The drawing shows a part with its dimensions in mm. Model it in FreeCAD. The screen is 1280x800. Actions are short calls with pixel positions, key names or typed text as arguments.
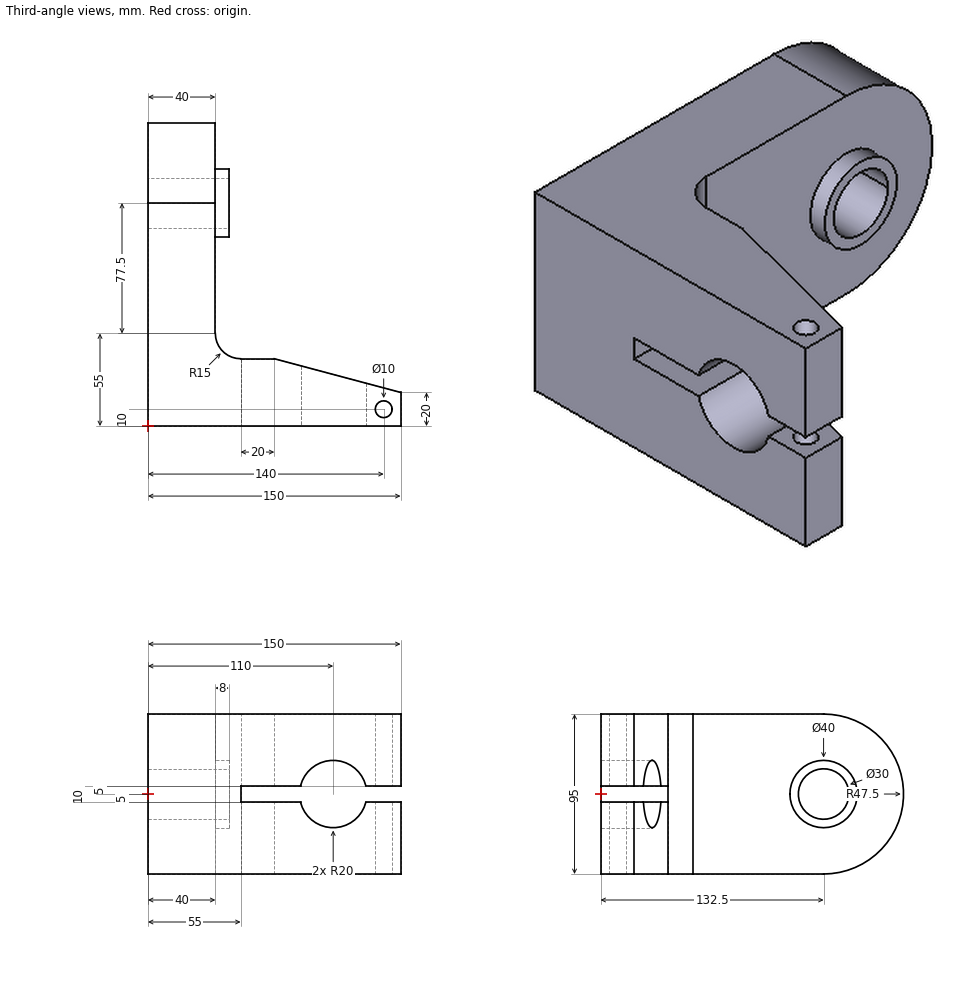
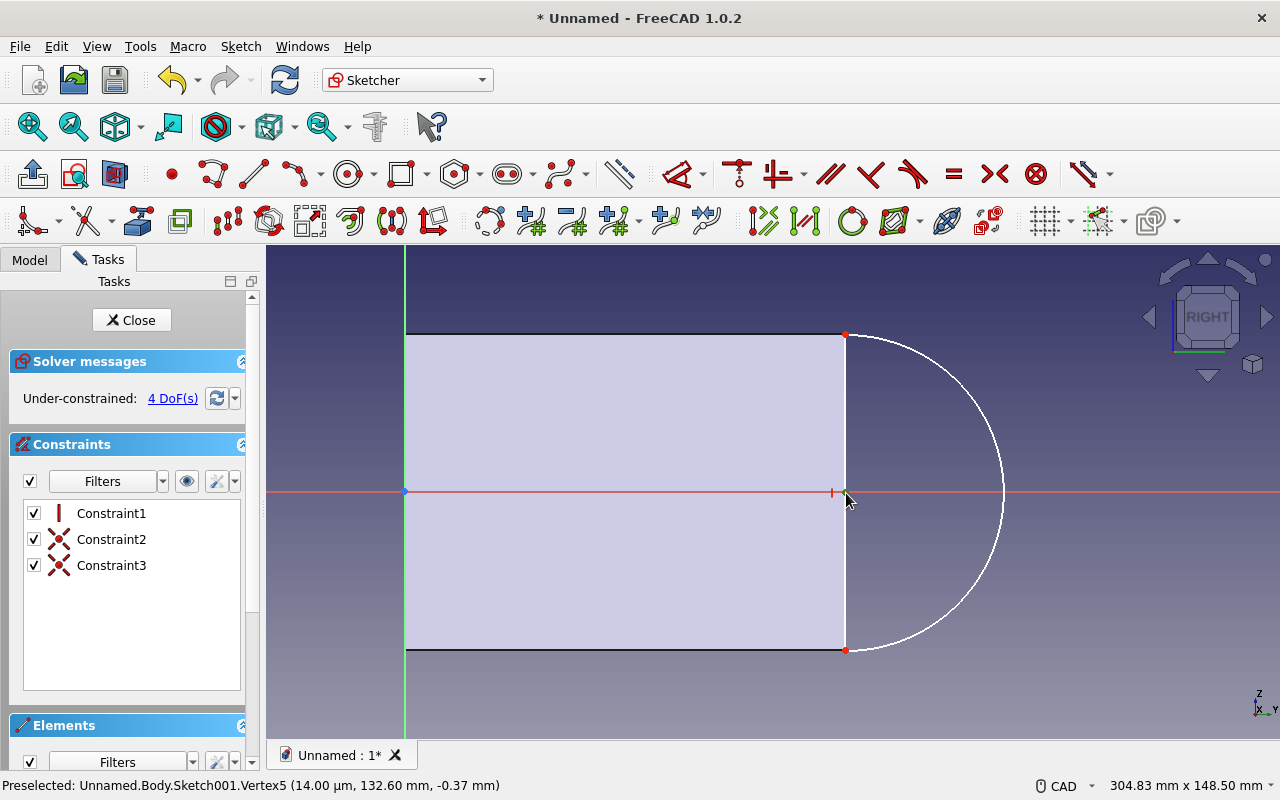
click(353, 492)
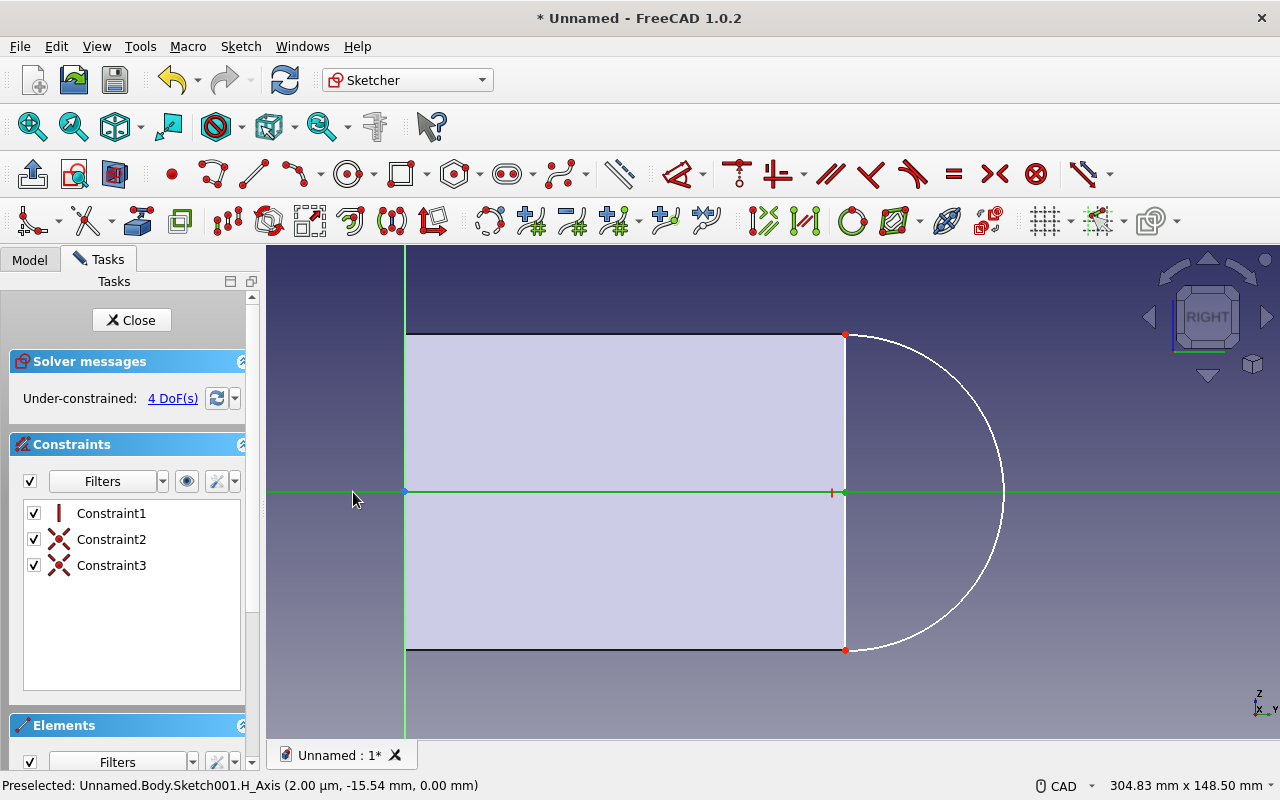
click(737, 174)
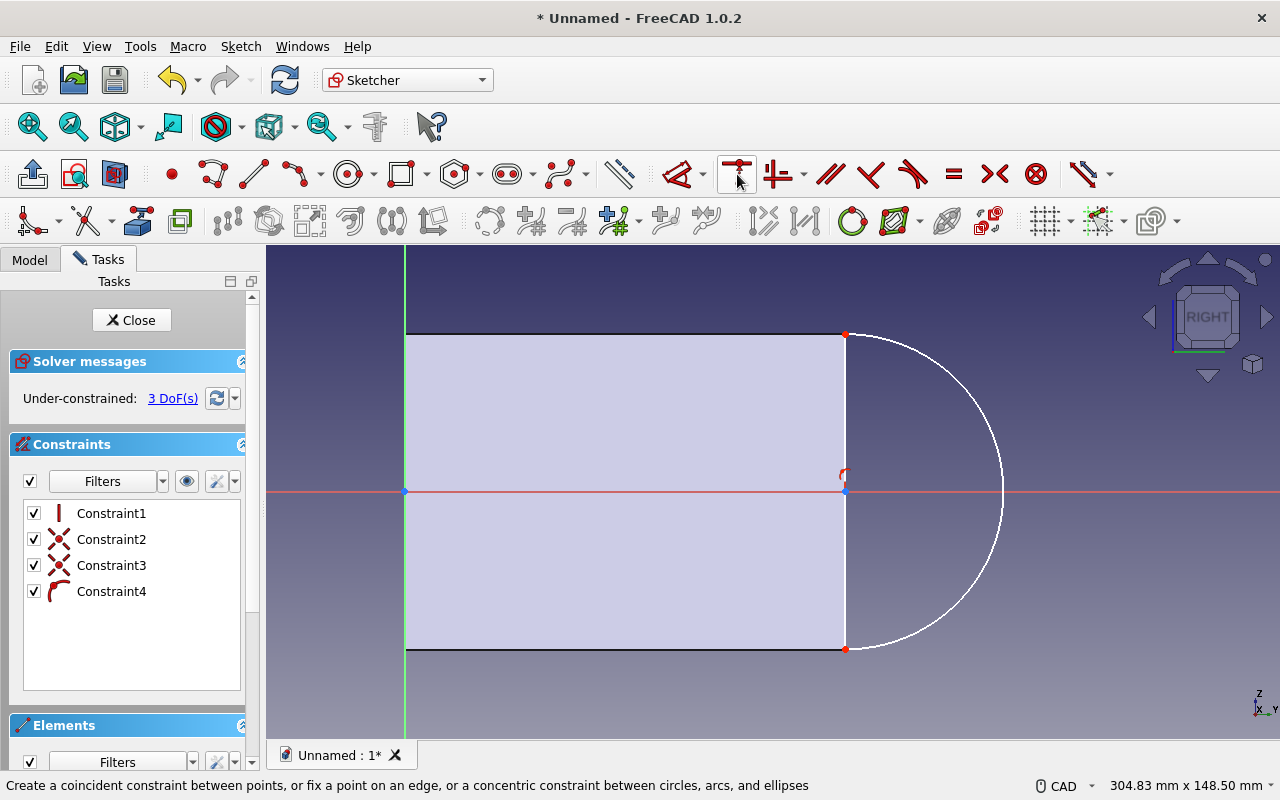
click(676, 174)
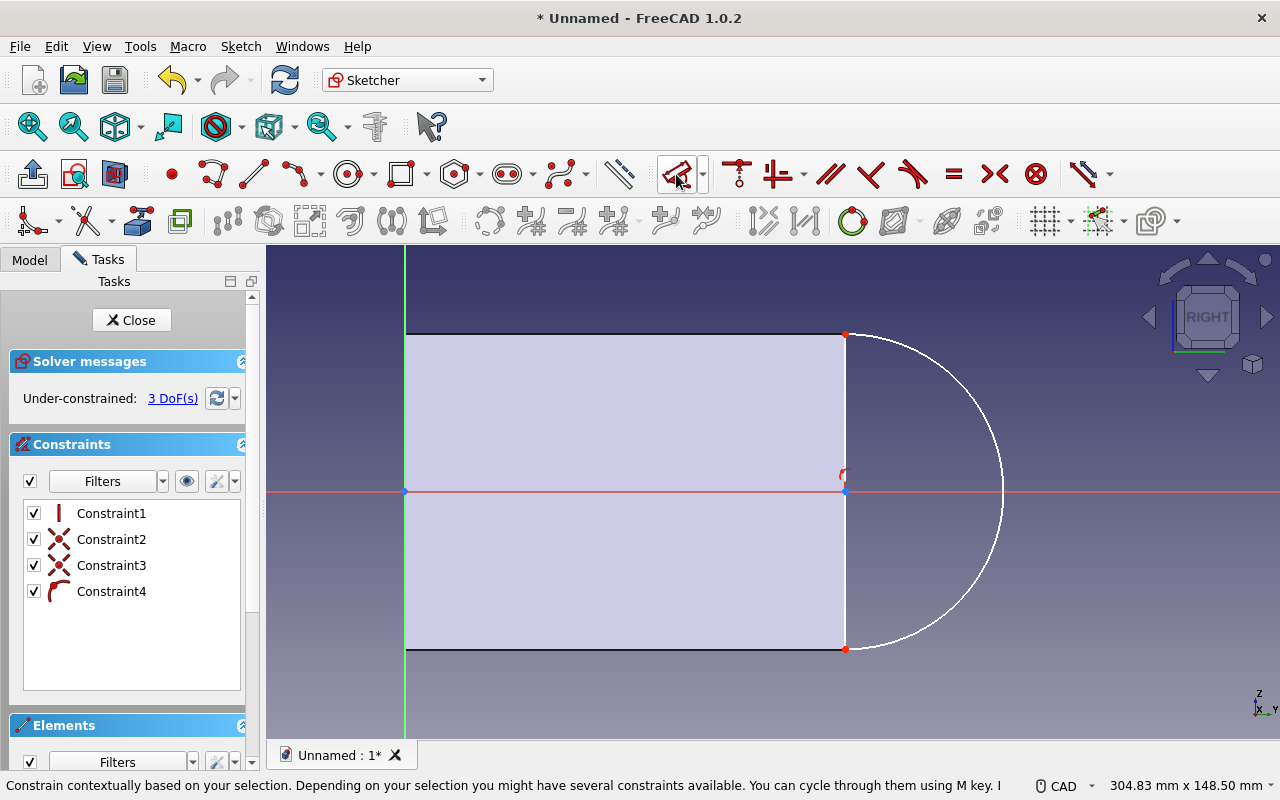
click(973, 585)
click(999, 604)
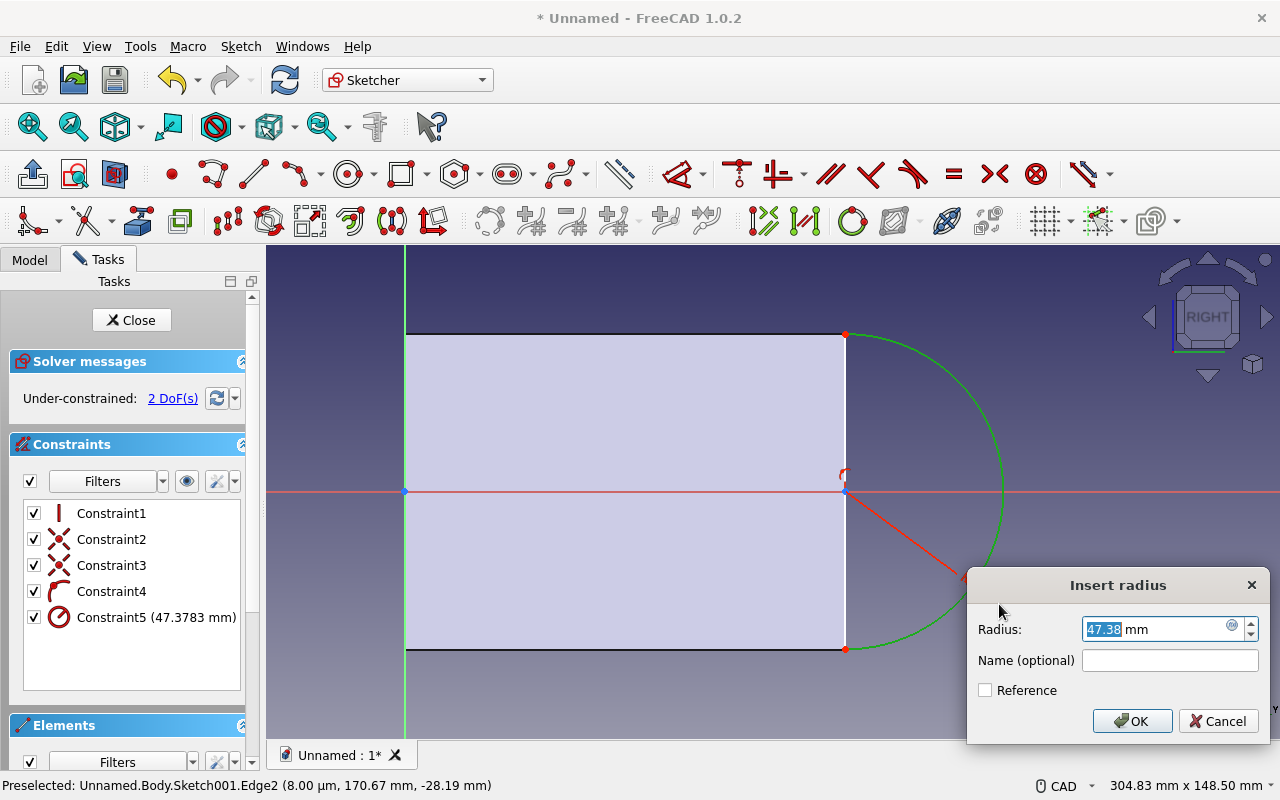
text(47.5)
key(Return)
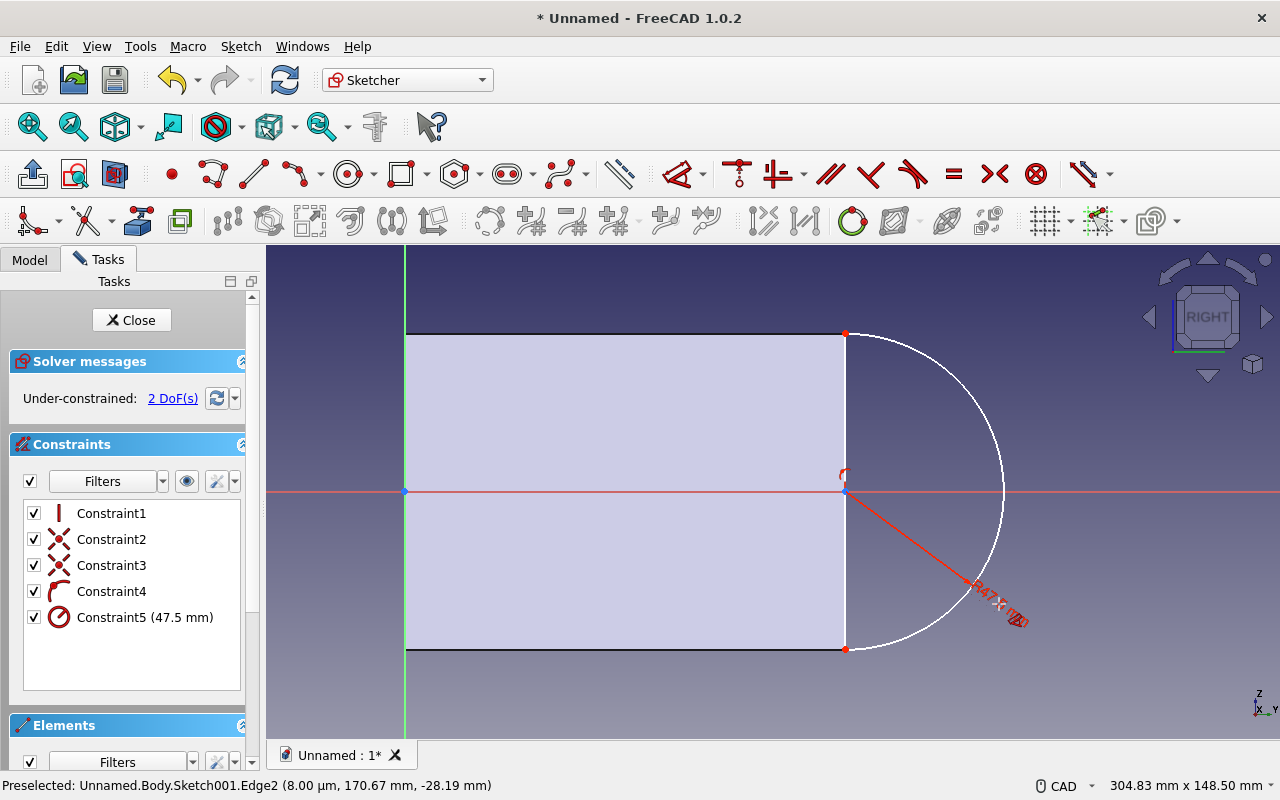
click(845, 650)
click(625, 684)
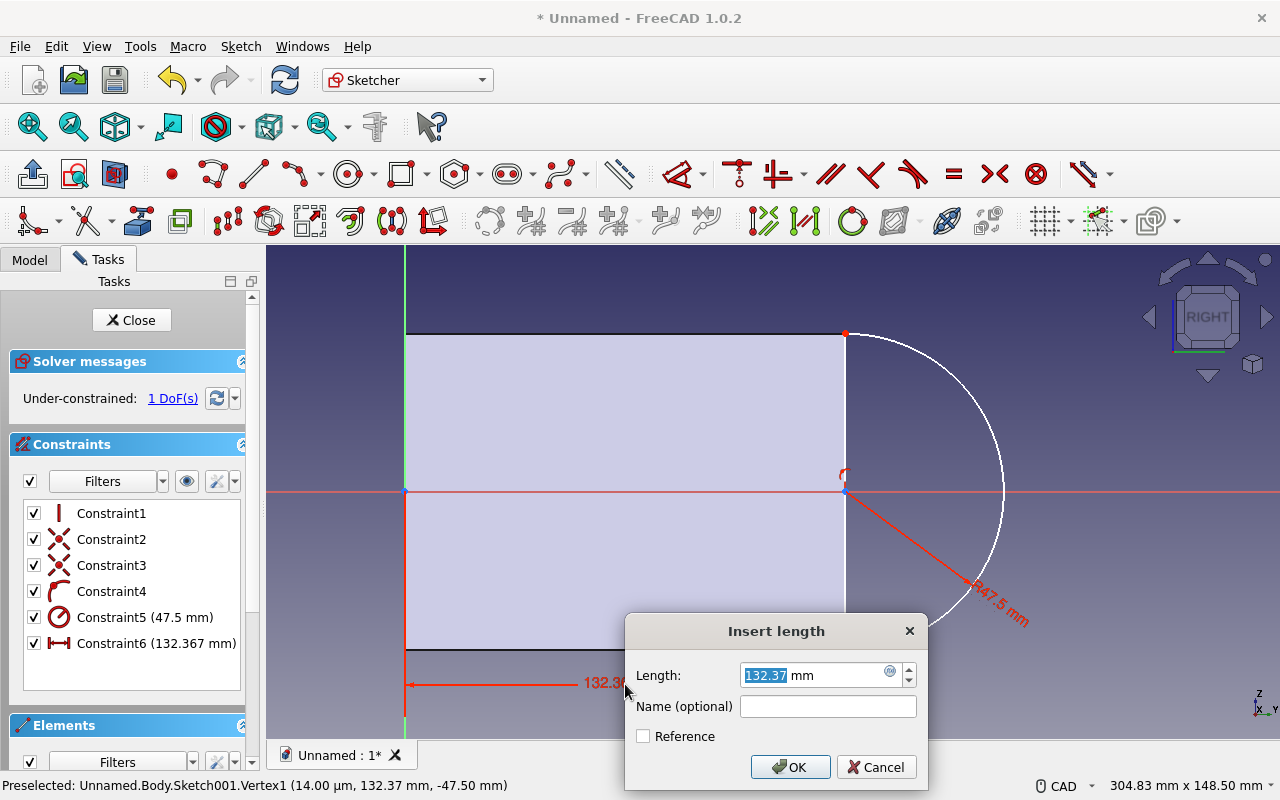
text(132.5)
key(Return)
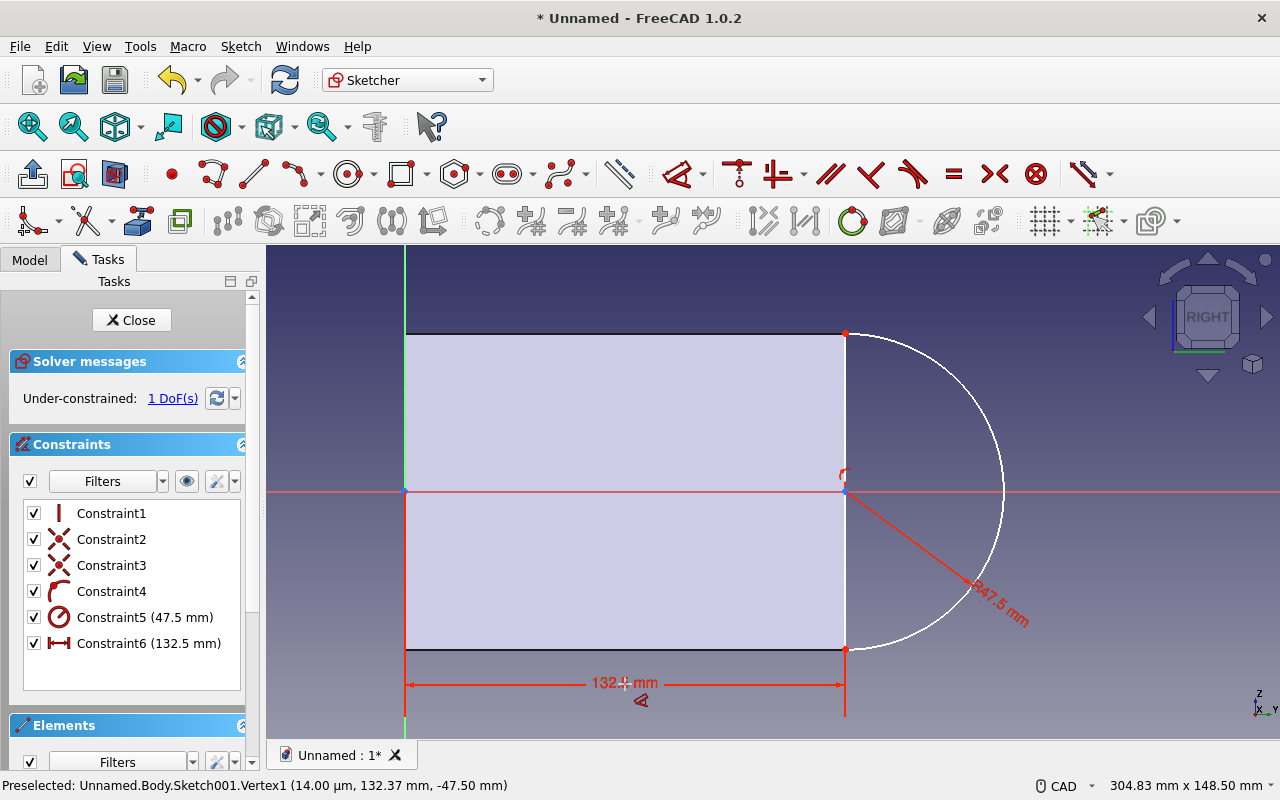
click(846, 492)
click(625, 526)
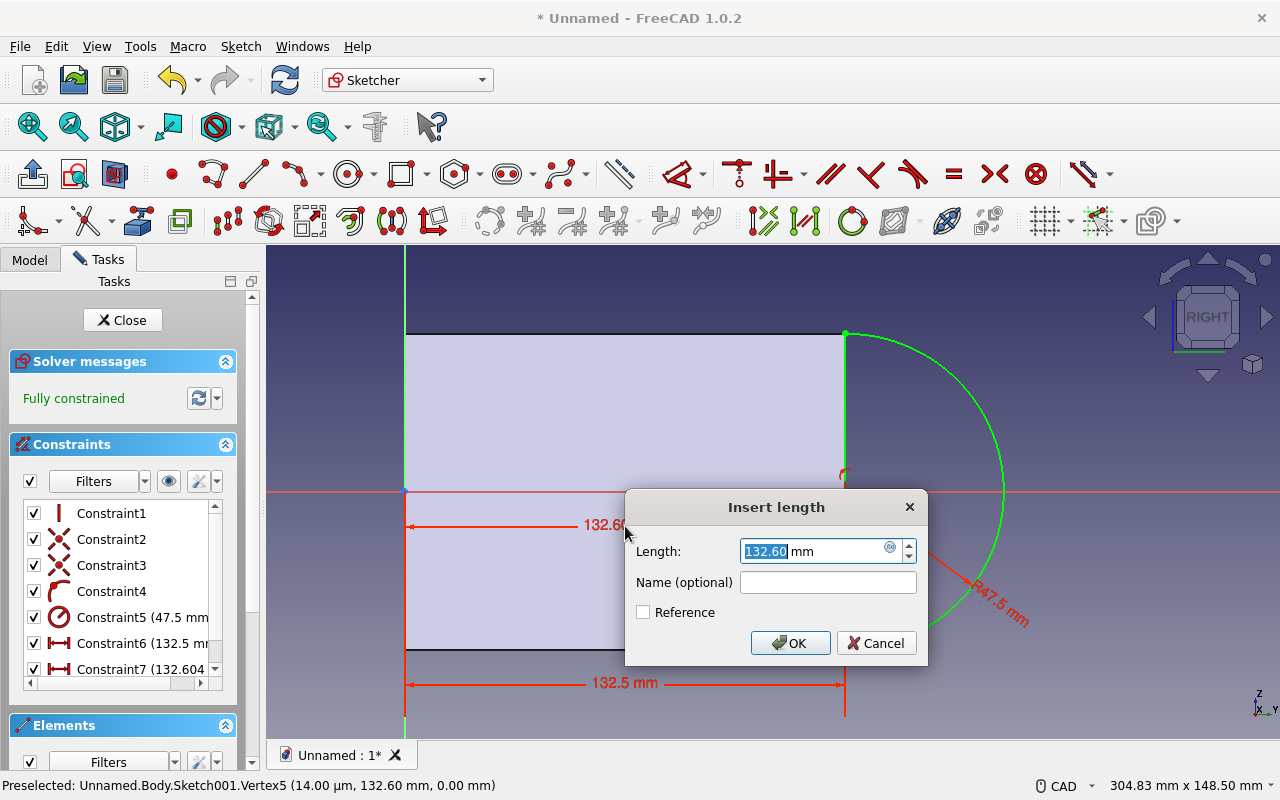
text(132.5)
key(Return)
key(Escape)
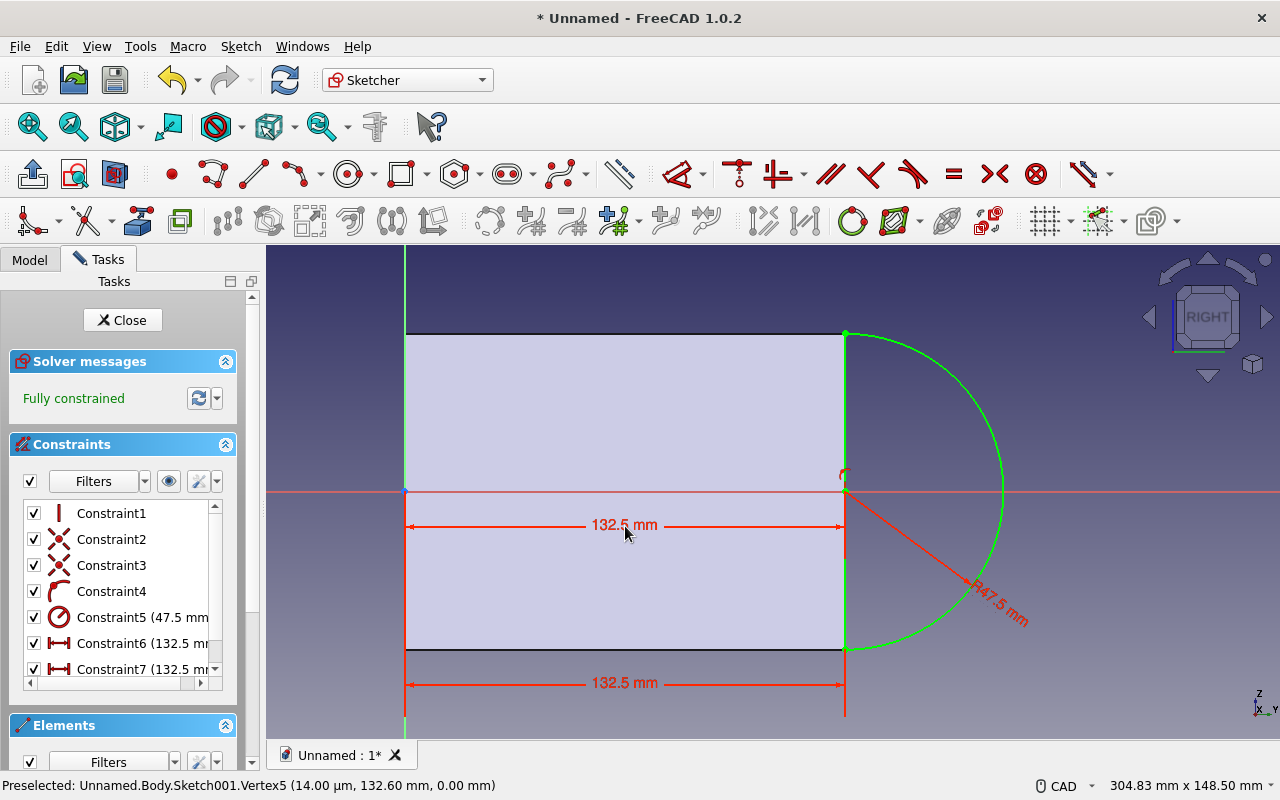
click(123, 320)